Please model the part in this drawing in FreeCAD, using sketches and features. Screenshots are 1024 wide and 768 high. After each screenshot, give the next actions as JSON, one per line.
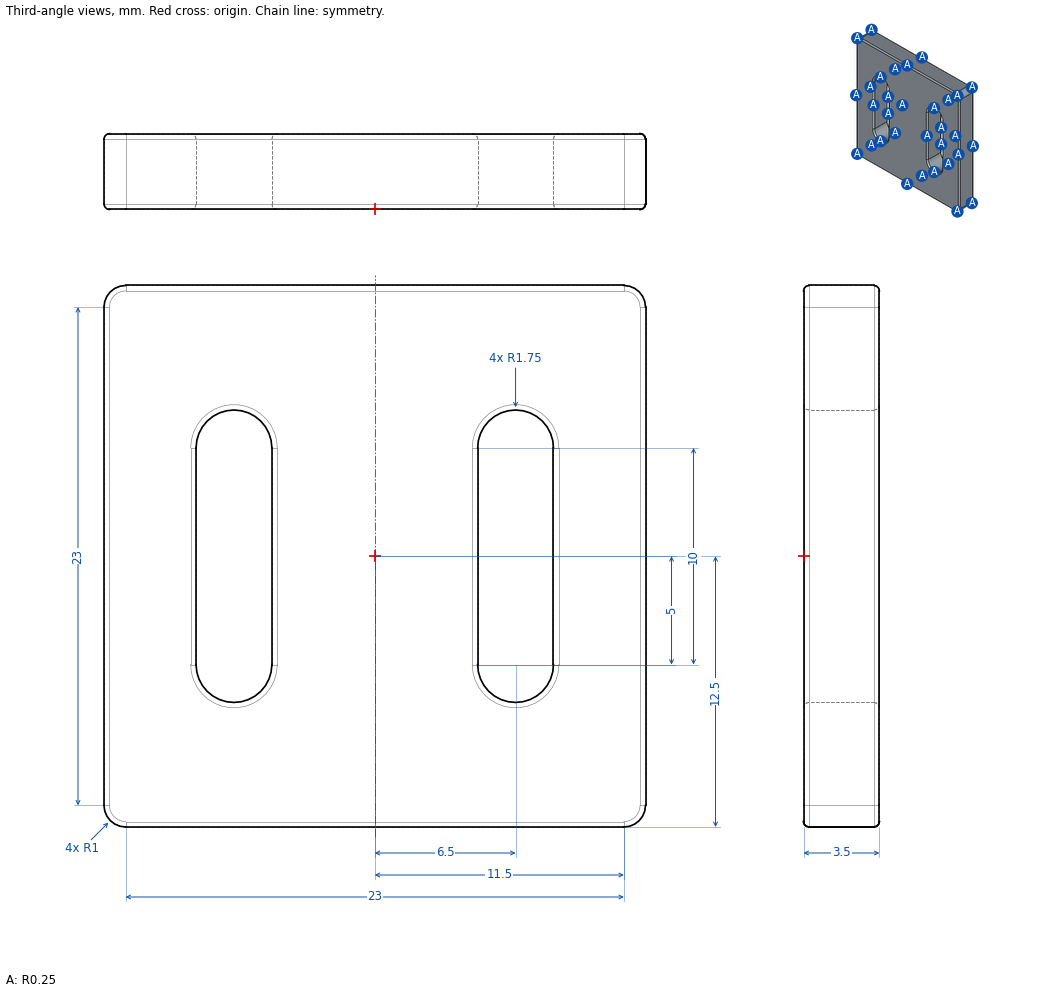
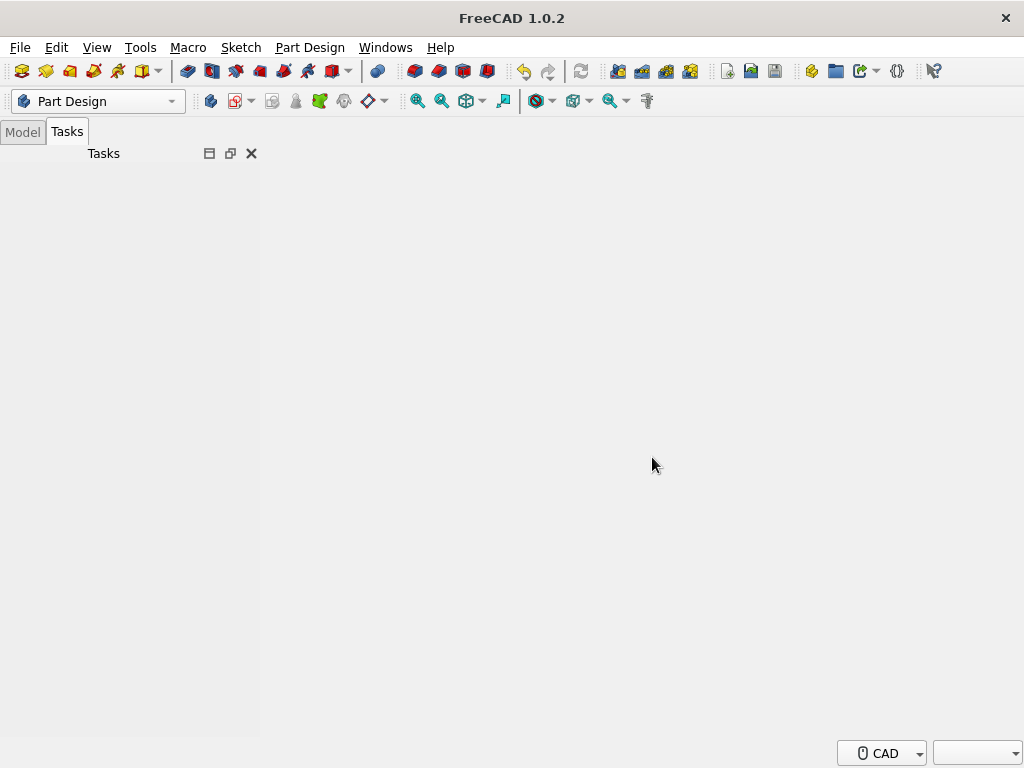
{"action": "key", "text": "ctrl+n"}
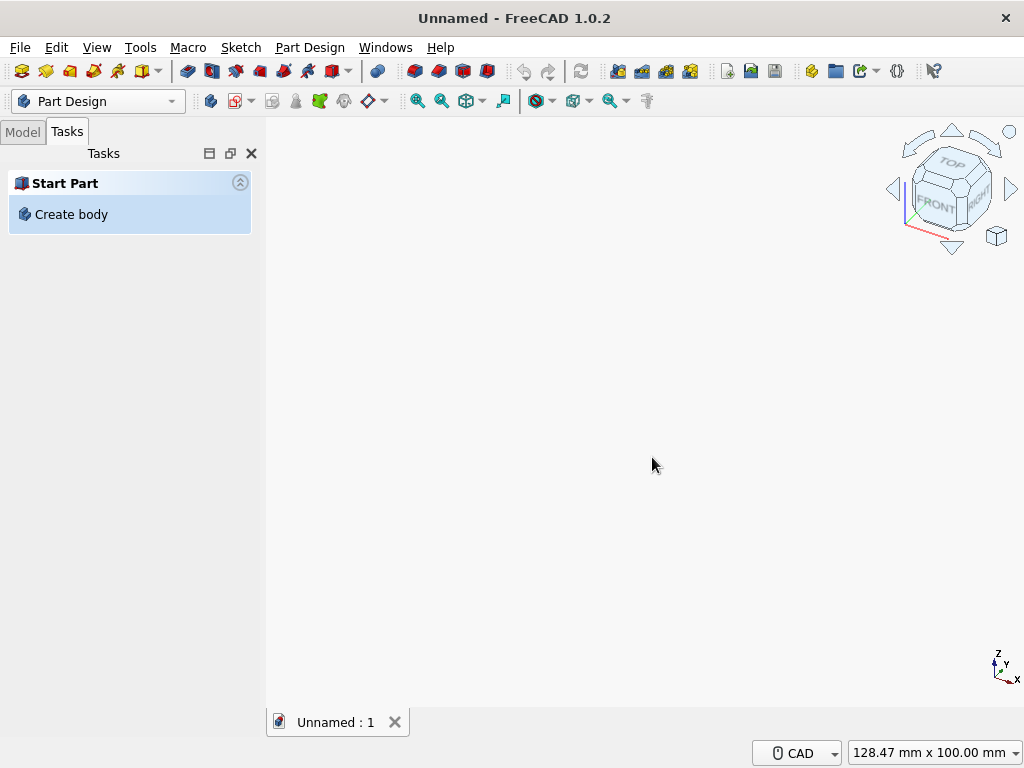
{"action": "left_click", "coordinate": [236, 102]}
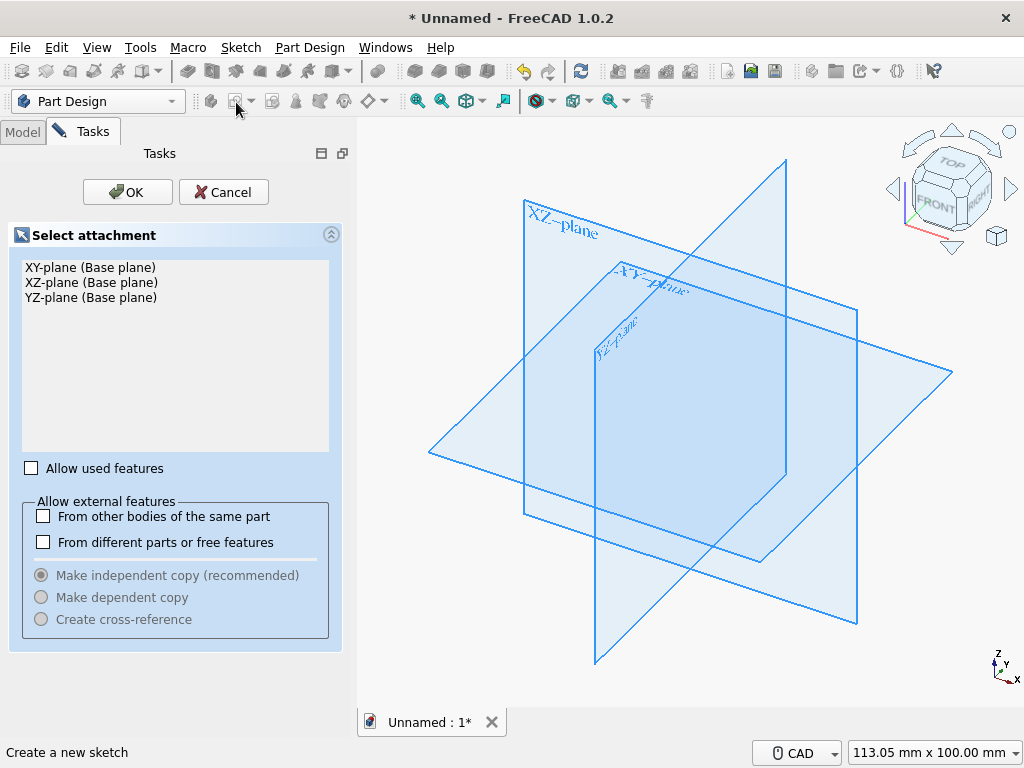
{"action": "left_click", "coordinate": [82, 282]}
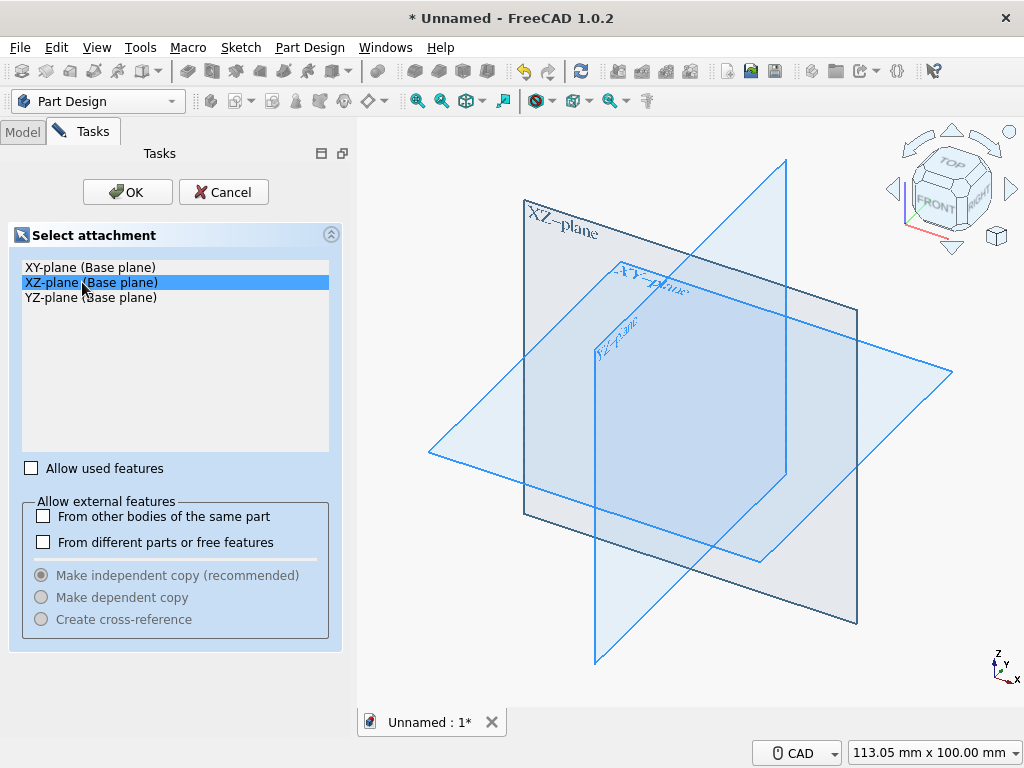
{"action": "left_click", "coordinate": [128, 192]}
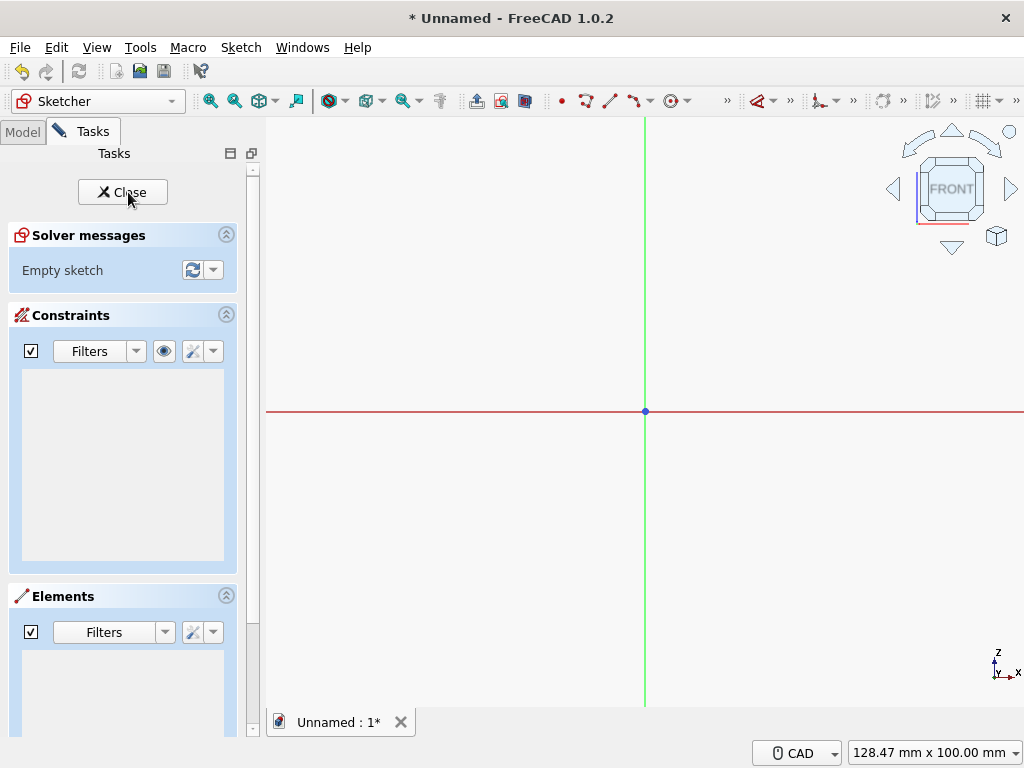
{"action": "scroll", "coordinate": [685, 412], "scroll_direction": "up", "scroll_amount": 5}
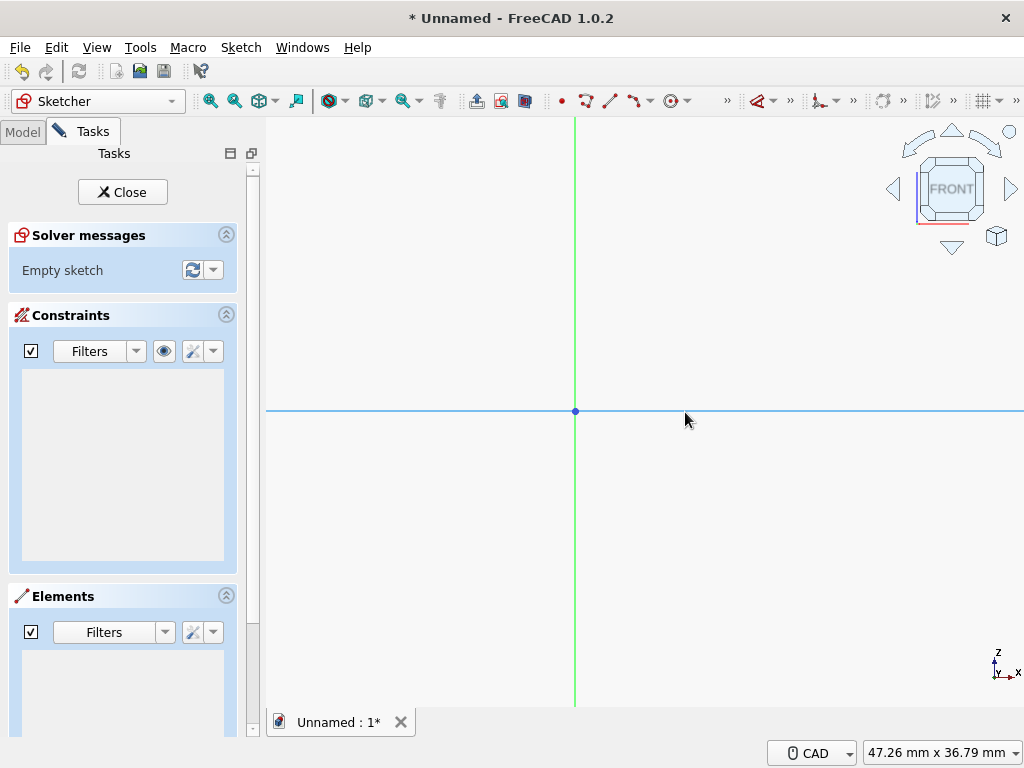
{"action": "left_click", "coordinate": [610, 102]}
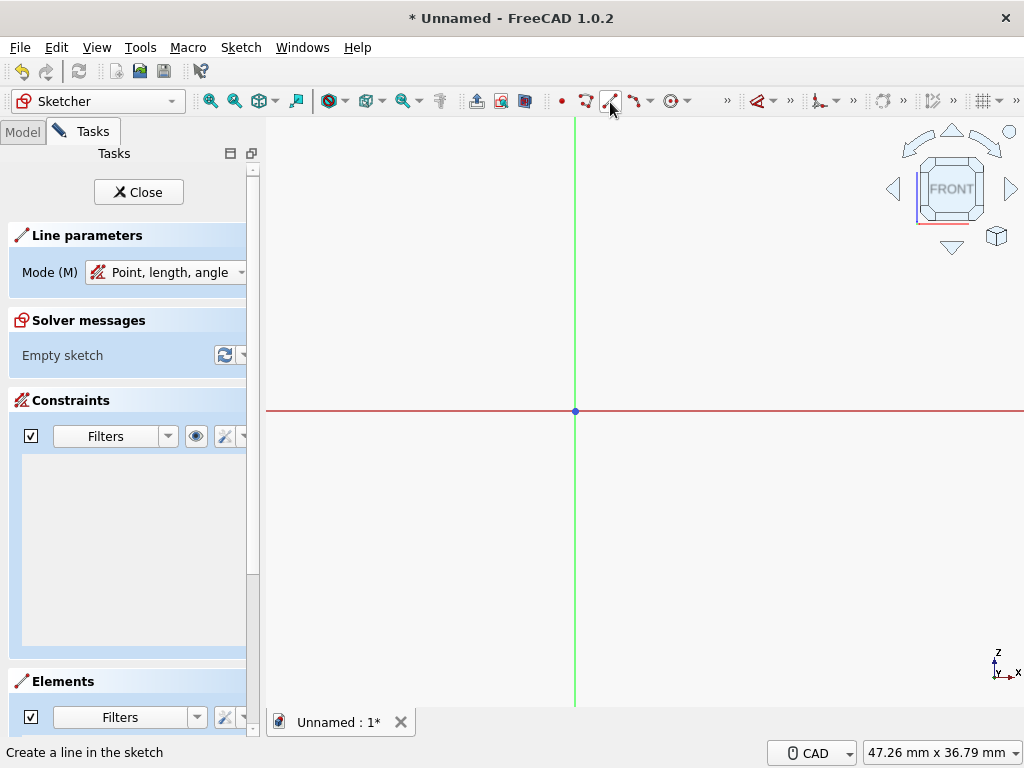
{"action": "left_click", "coordinate": [760, 612]}
{"action": "left_click", "coordinate": [391, 612]}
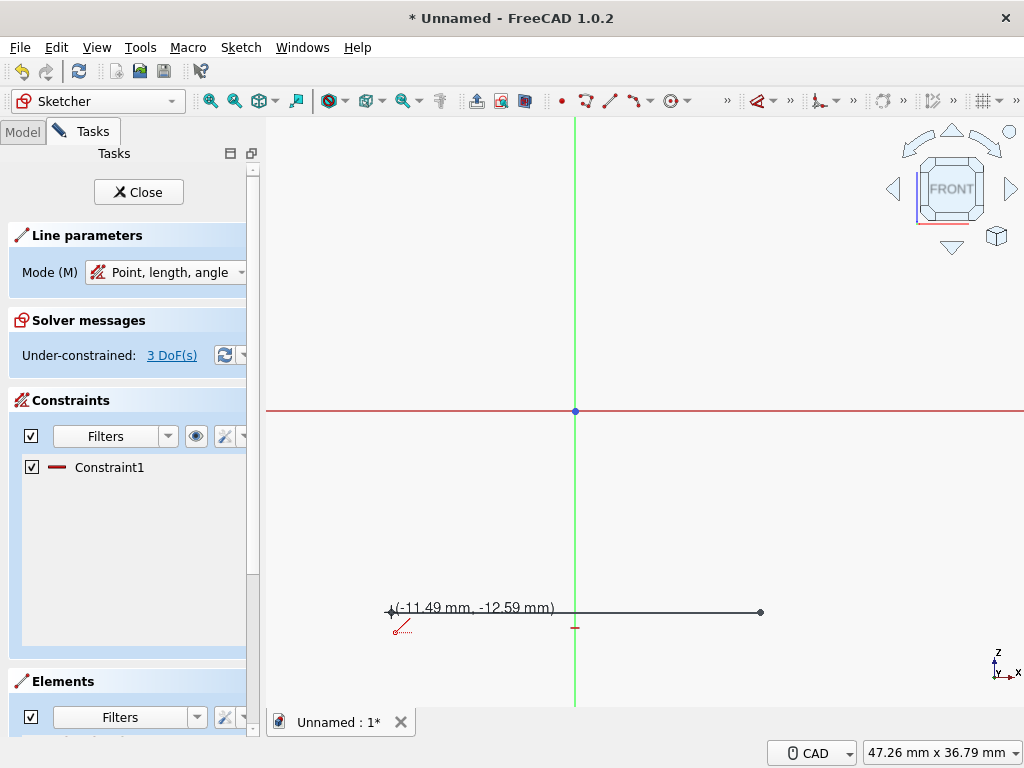
{"action": "left_click", "coordinate": [375, 596]}
{"action": "left_click", "coordinate": [375, 227]}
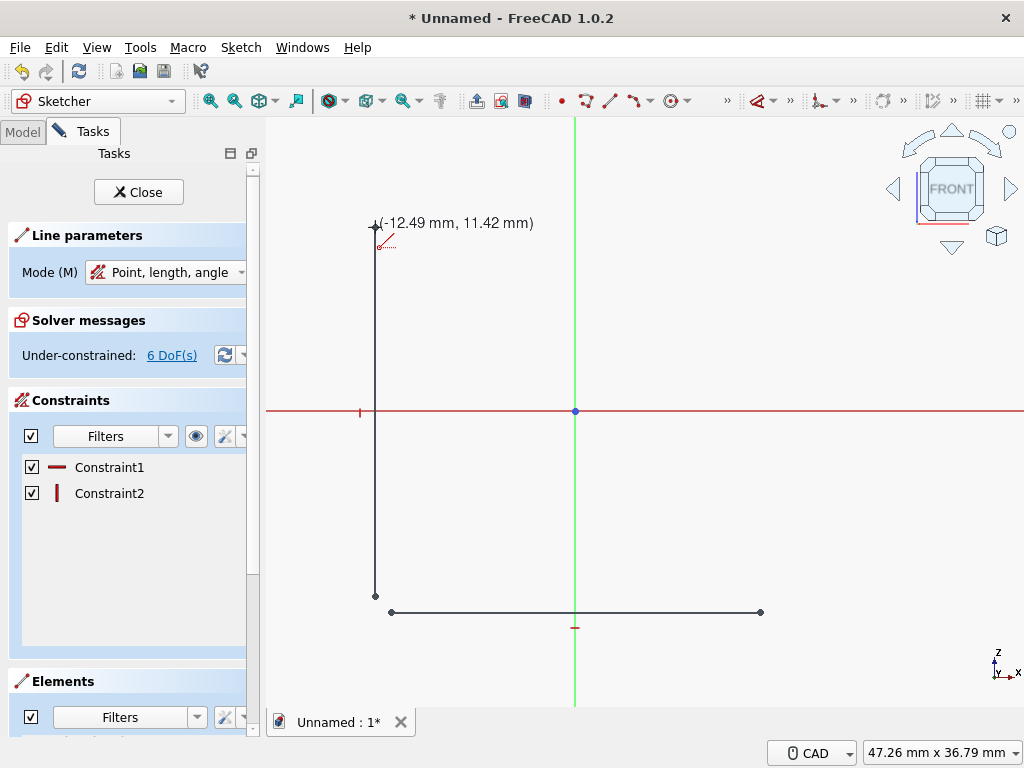
{"action": "left_click", "coordinate": [391, 211]}
{"action": "left_click", "coordinate": [760, 211]}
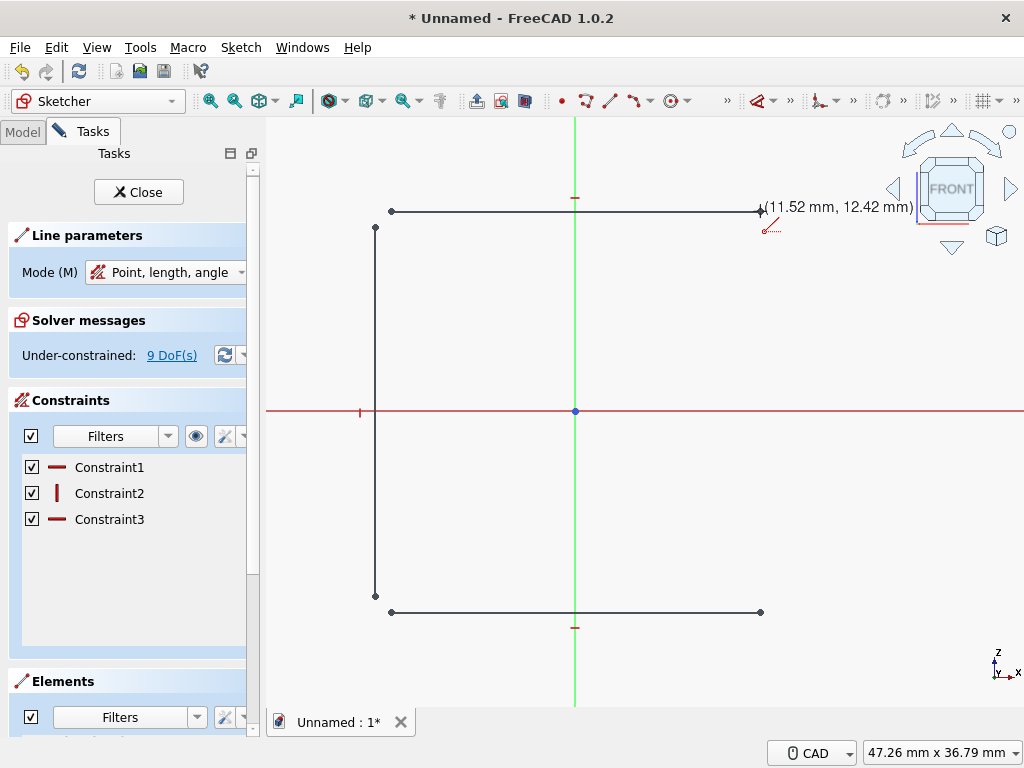
{"action": "left_click", "coordinate": [776, 227]}
{"action": "left_click", "coordinate": [776, 596]}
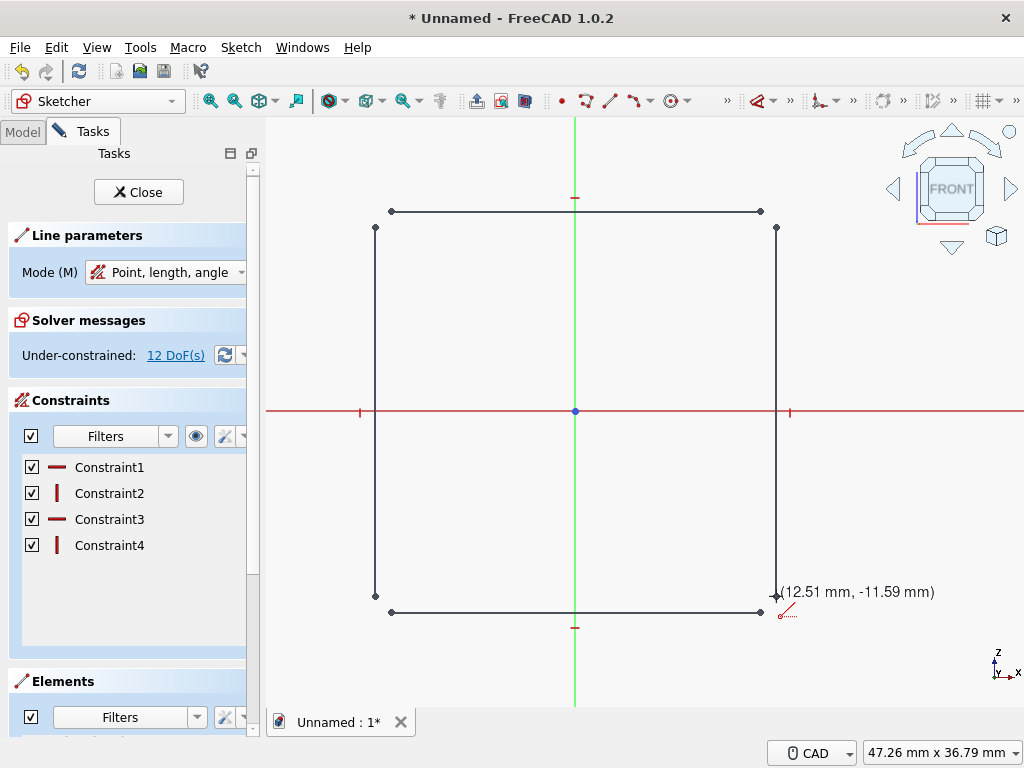
{"action": "left_click", "coordinate": [634, 102]}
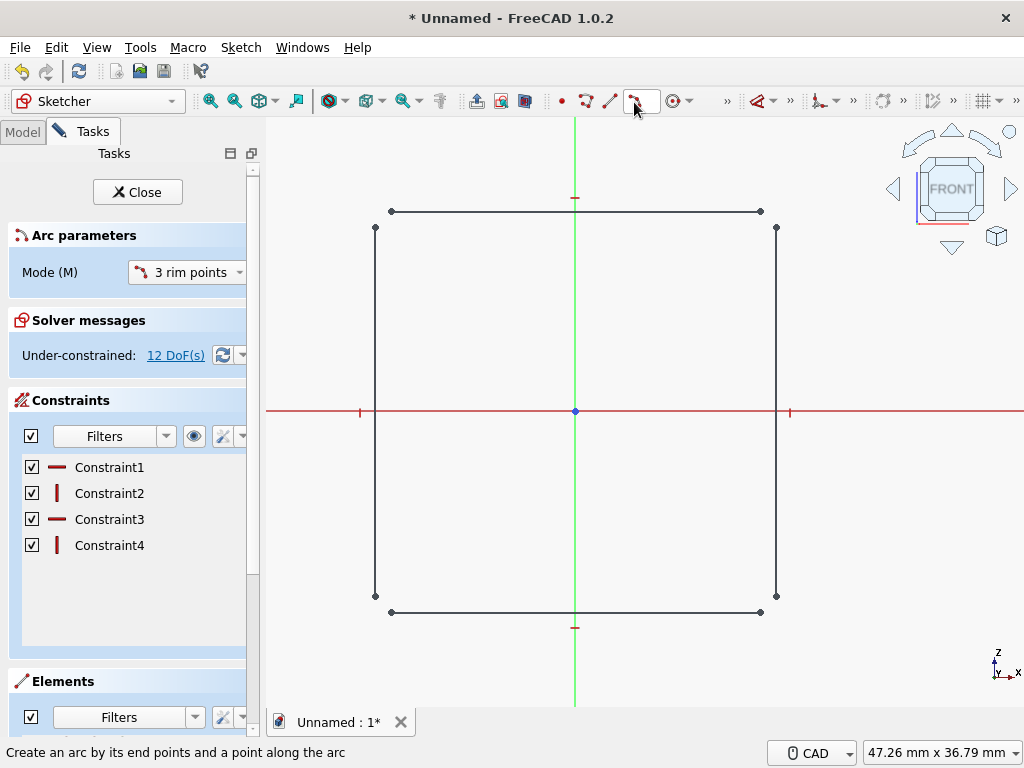
{"action": "left_click", "coordinate": [391, 613]}
{"action": "left_click", "coordinate": [375, 597]}